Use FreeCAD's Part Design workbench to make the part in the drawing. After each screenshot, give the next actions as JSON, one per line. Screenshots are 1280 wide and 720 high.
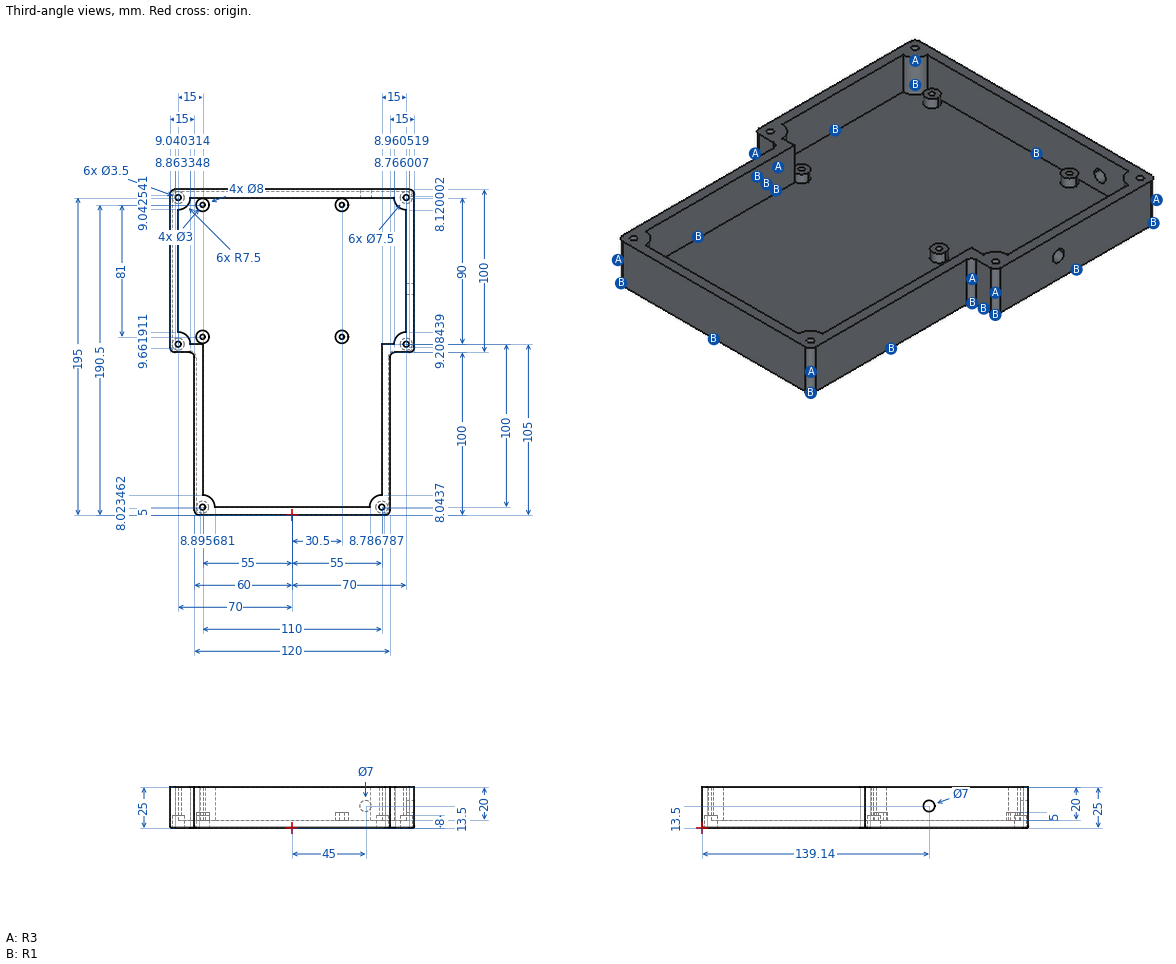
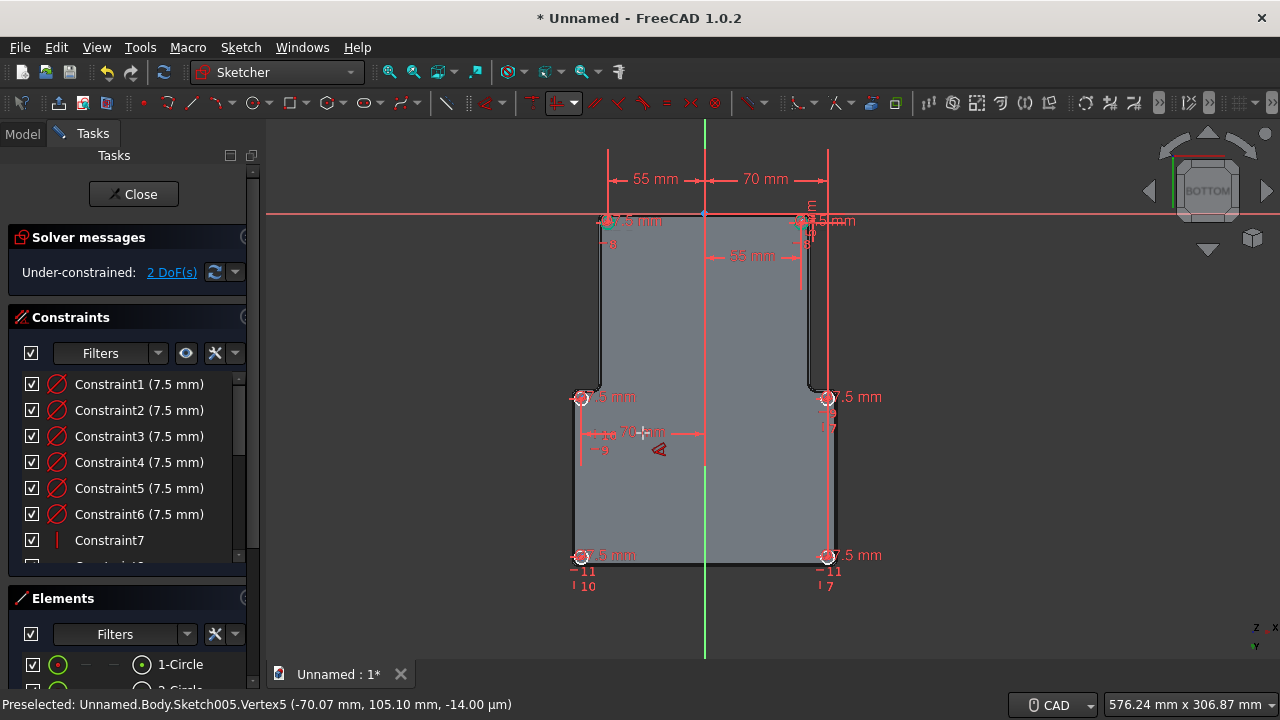
{"action": "left_click", "coordinate": [828, 557]}
{"action": "left_click", "coordinate": [862, 386]}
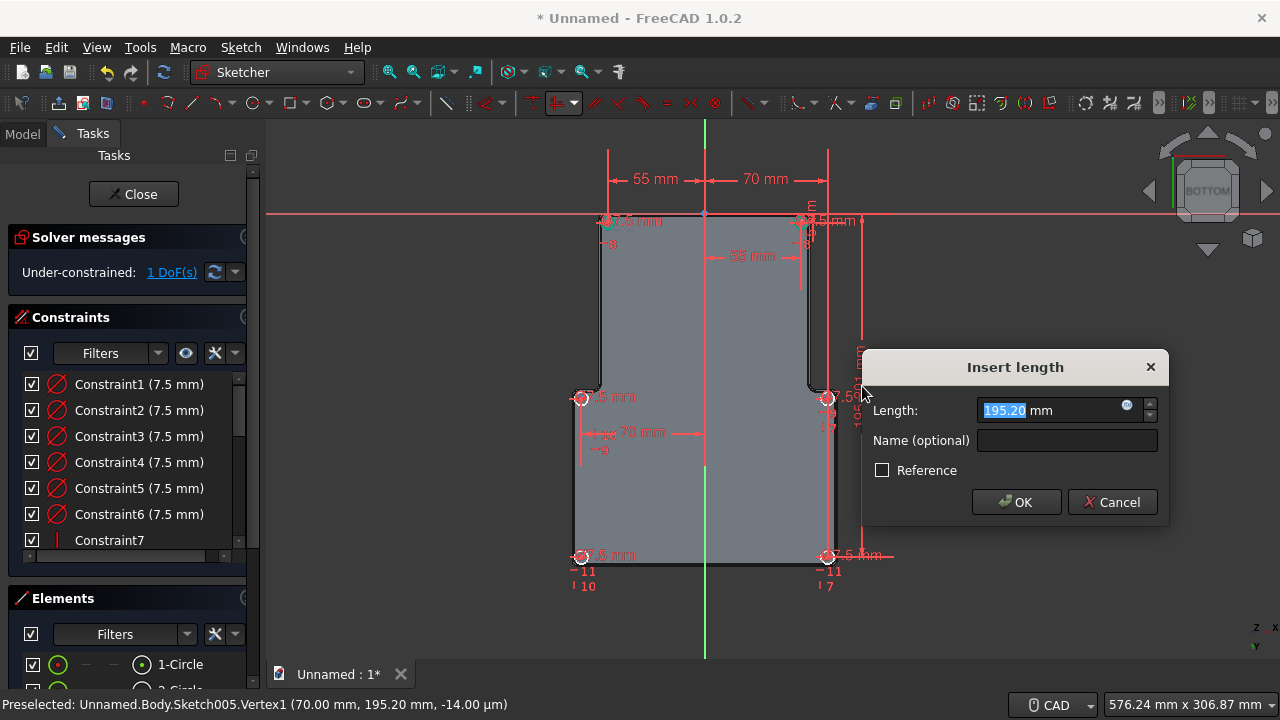
{"action": "type", "text": "195"}
{"action": "key", "text": "Return"}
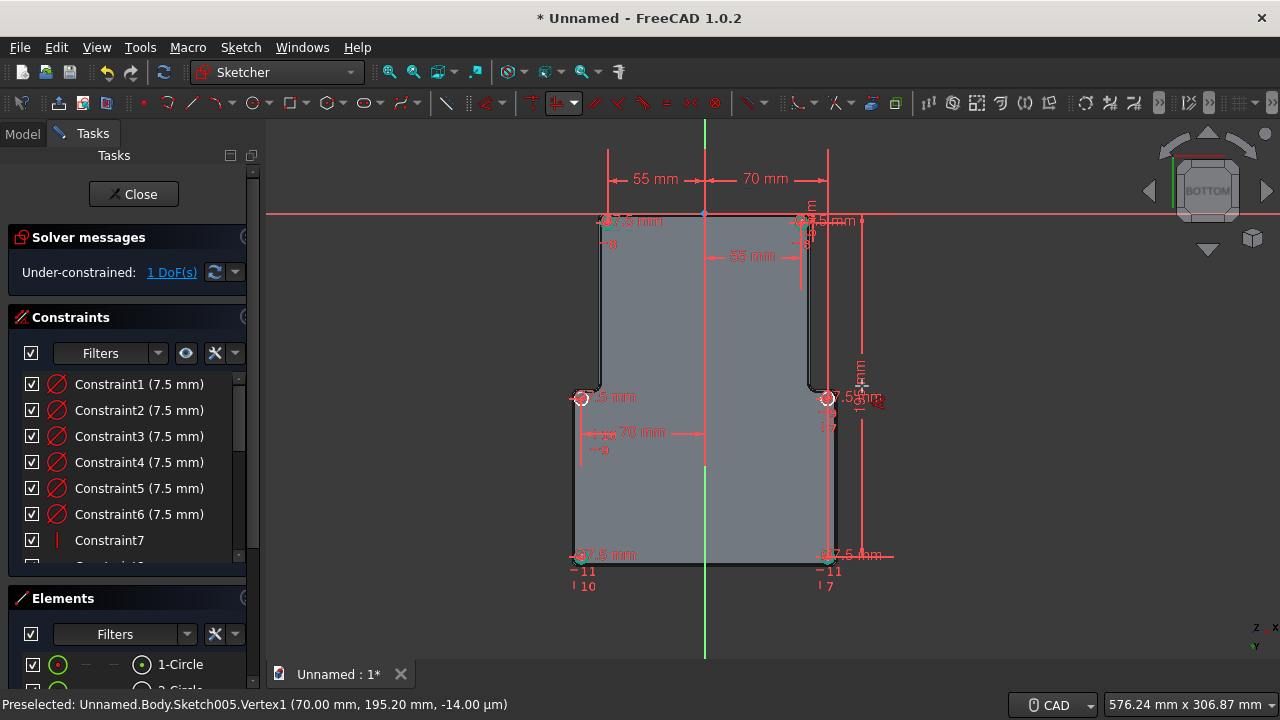
{"action": "left_click", "coordinate": [828, 399]}
{"action": "left_click", "coordinate": [862, 306]}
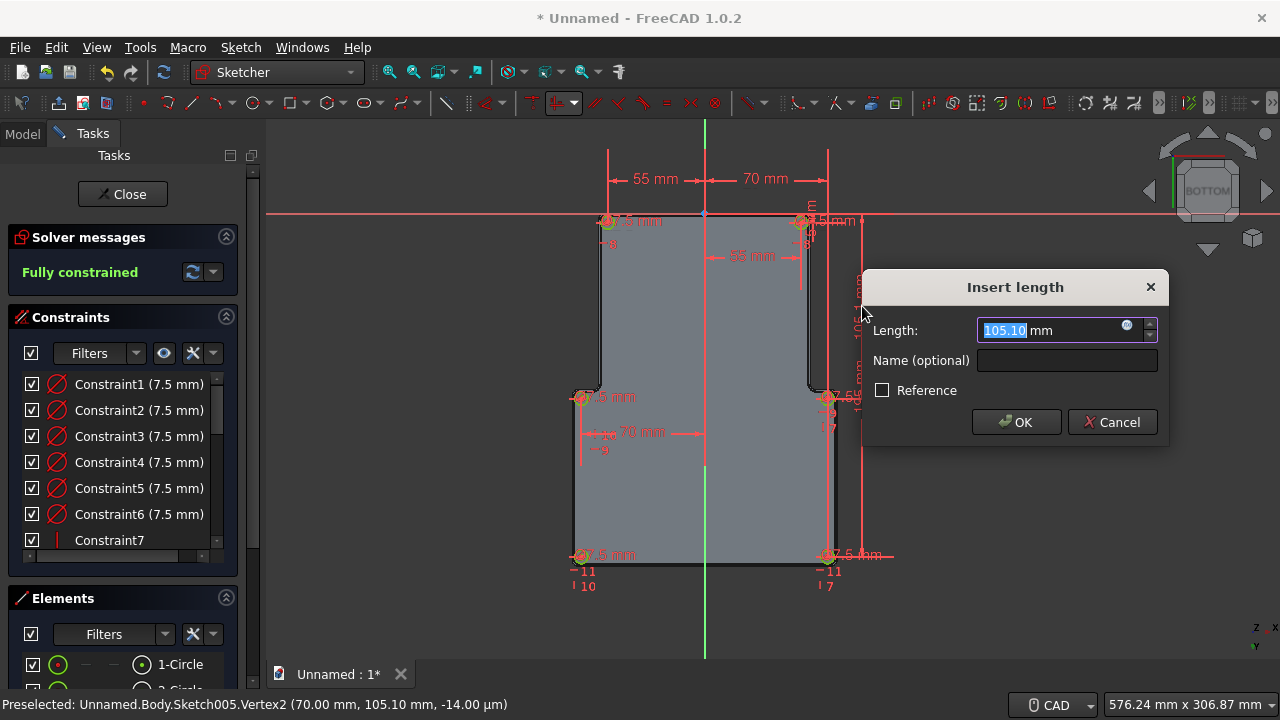
{"action": "type", "text": "105"}
{"action": "key", "text": "Return"}
{"action": "key", "text": "Escape"}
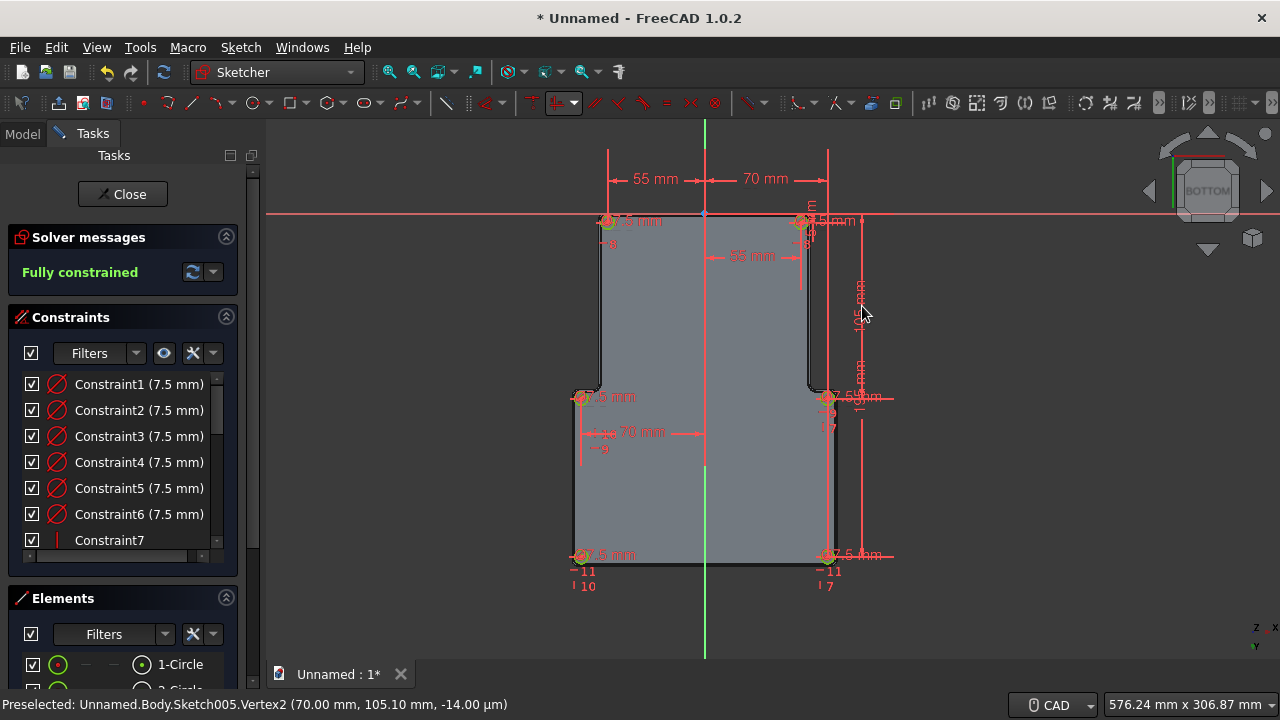
{"action": "left_click", "coordinate": [123, 194]}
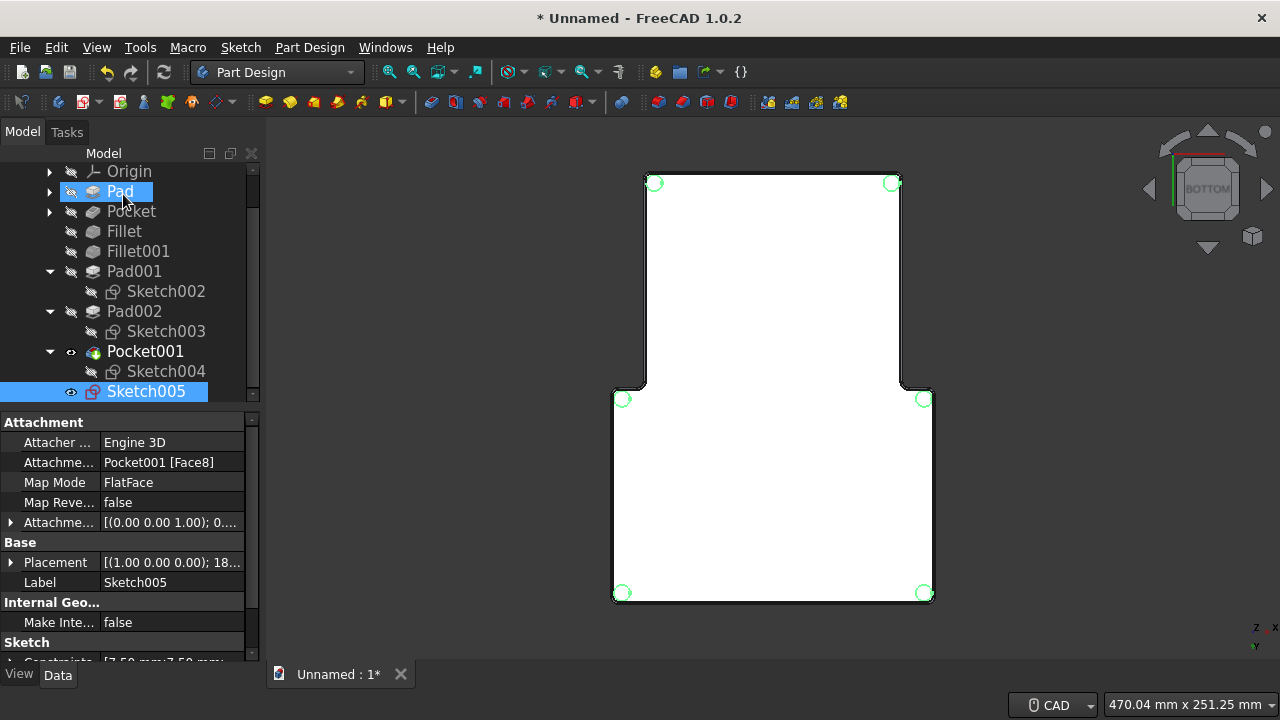
{"action": "left_click", "coordinate": [432, 102]}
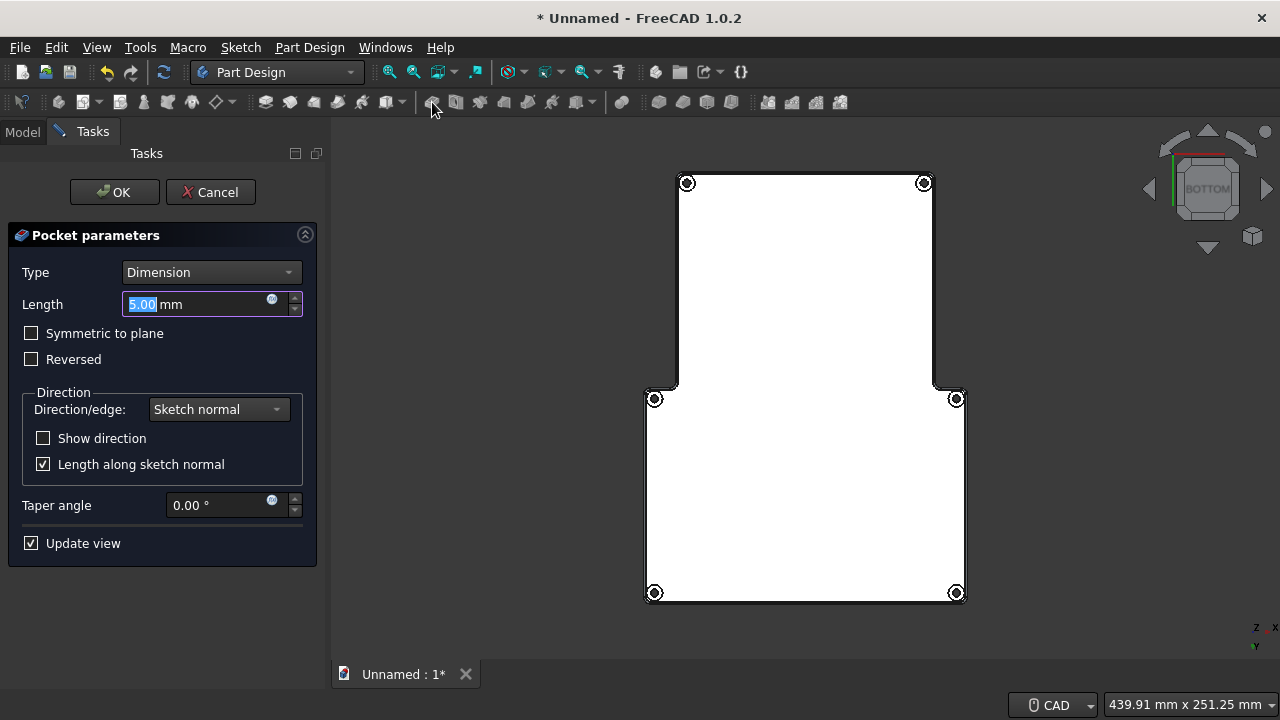
{"action": "type", "text": "8"}
{"action": "key", "text": "Tab"}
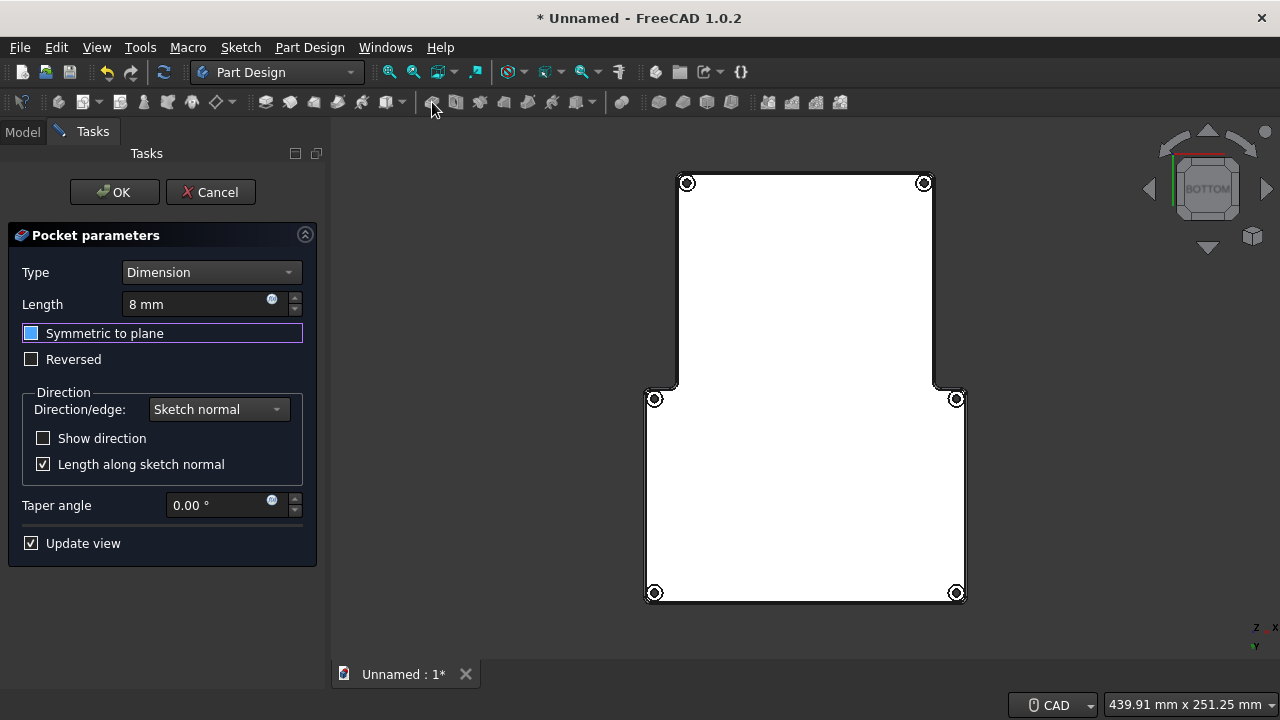
{"action": "left_click", "coordinate": [115, 192]}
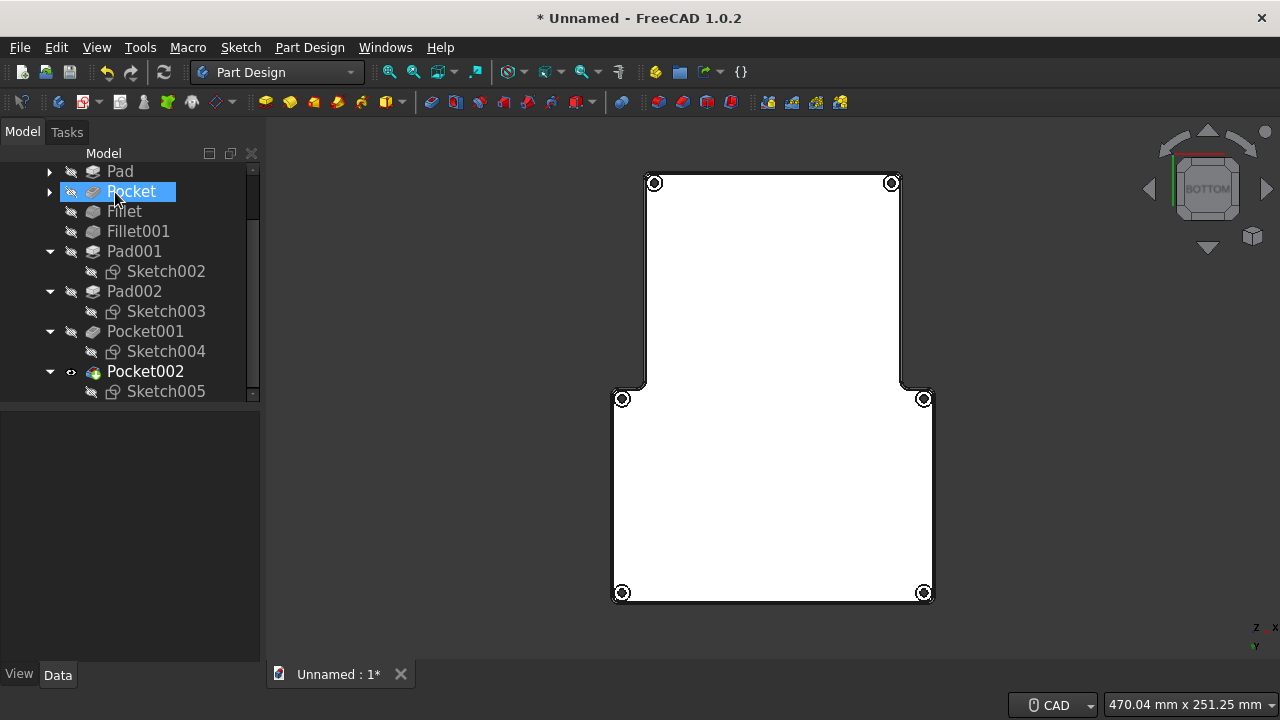
{"action": "key", "text": "0"}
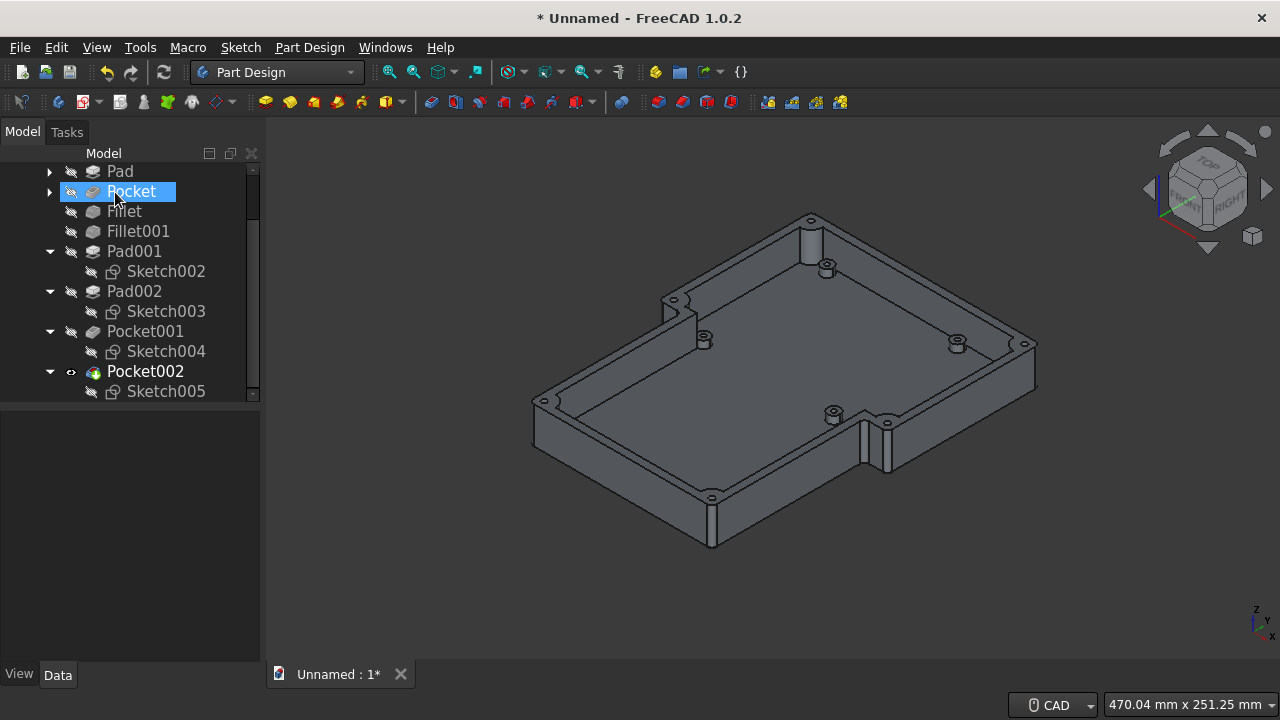
{"action": "left_click", "coordinate": [1005, 384]}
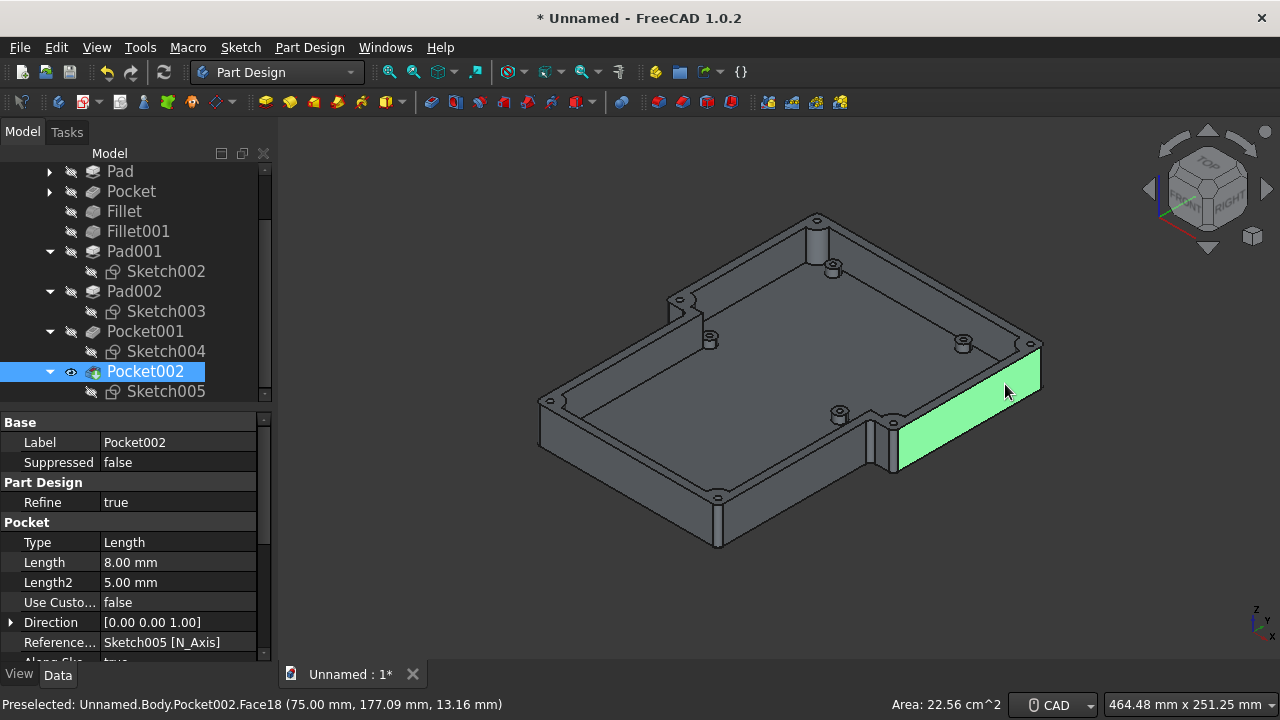
{"action": "left_click", "coordinate": [84, 102]}